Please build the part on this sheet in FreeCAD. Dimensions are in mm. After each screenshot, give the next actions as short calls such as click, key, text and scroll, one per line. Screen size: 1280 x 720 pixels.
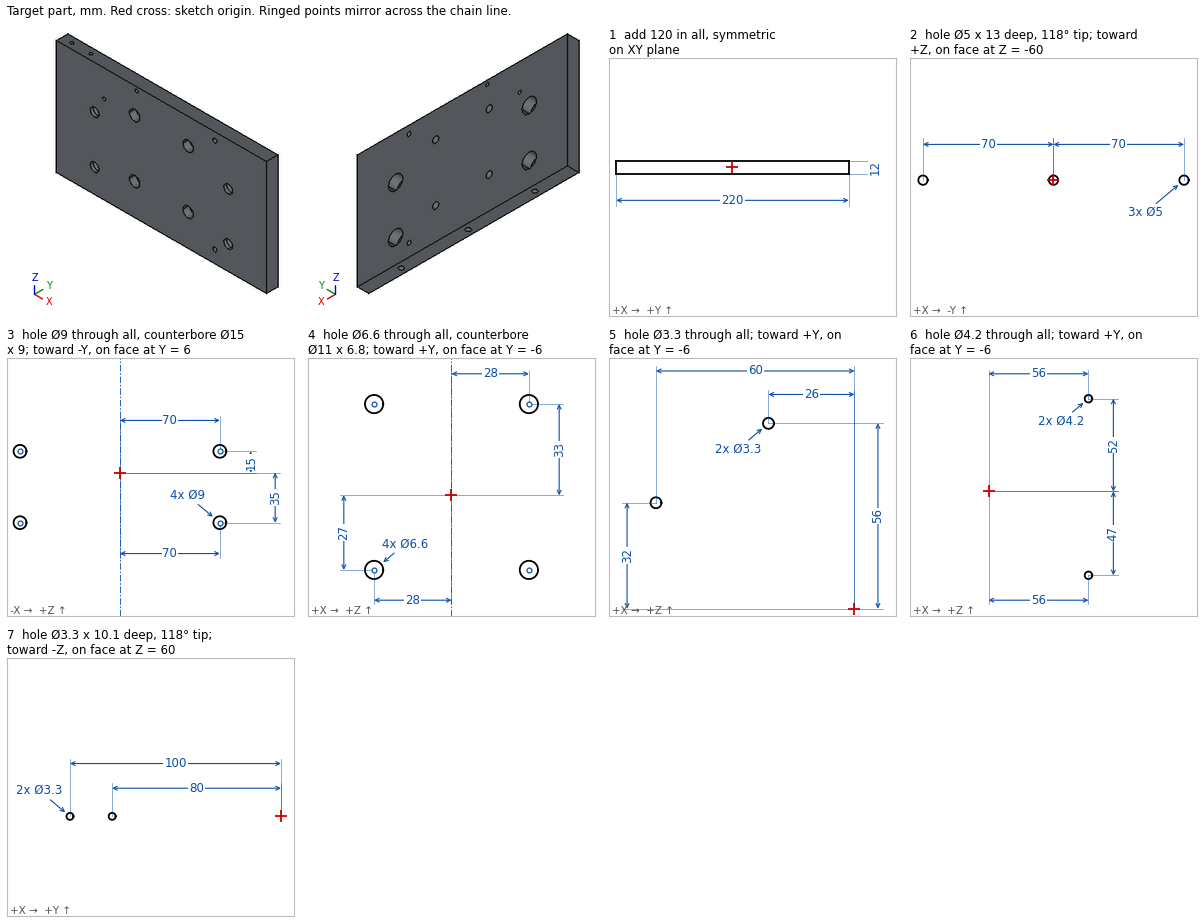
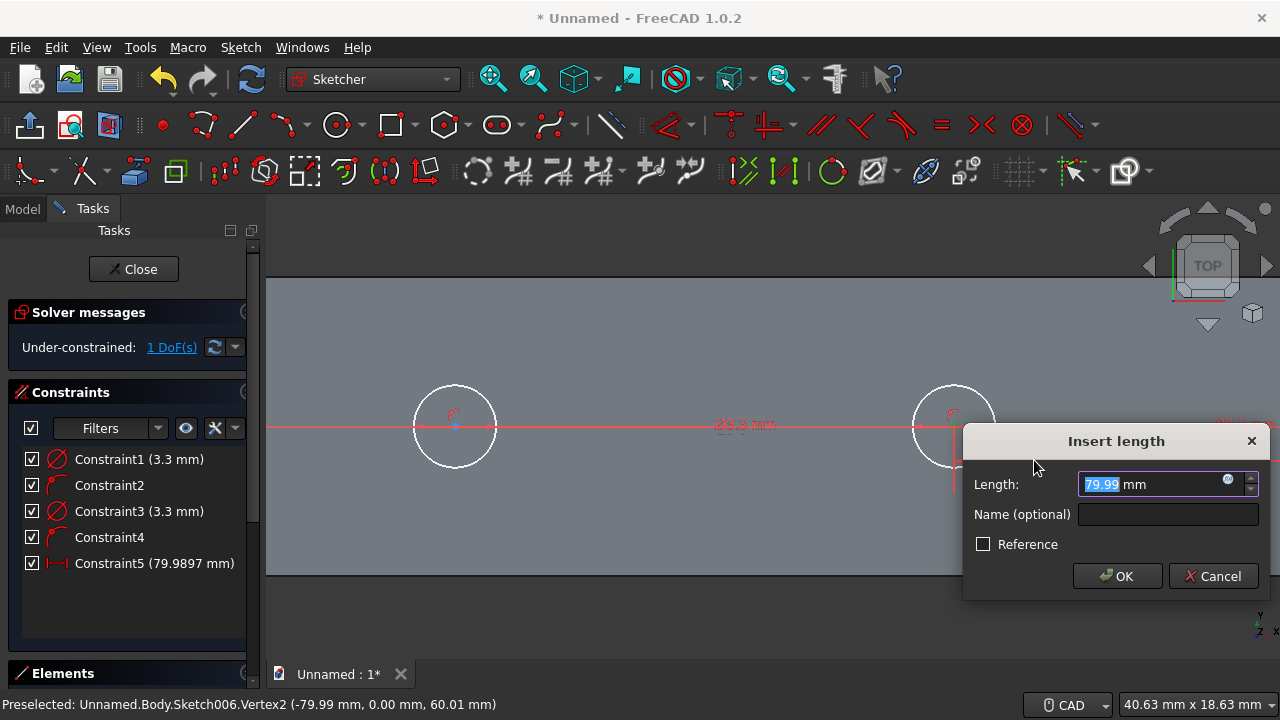
text(80)
key(Return)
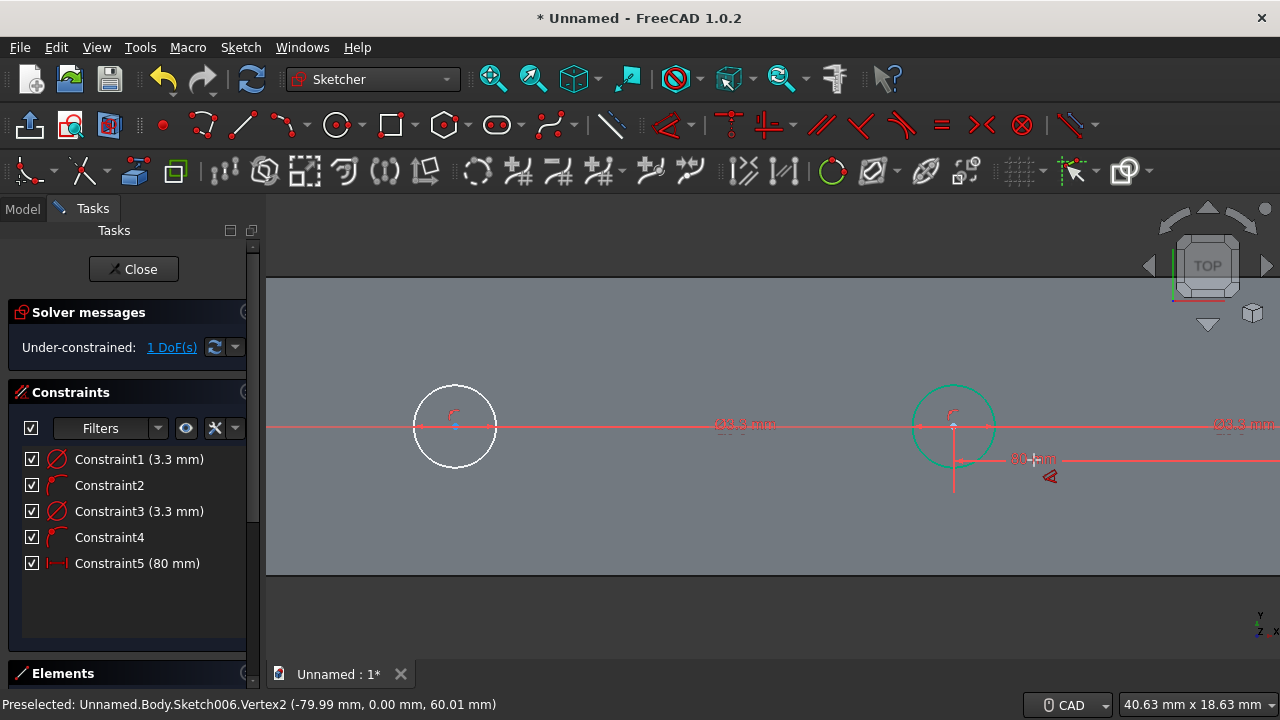
click(455, 426)
click(785, 460)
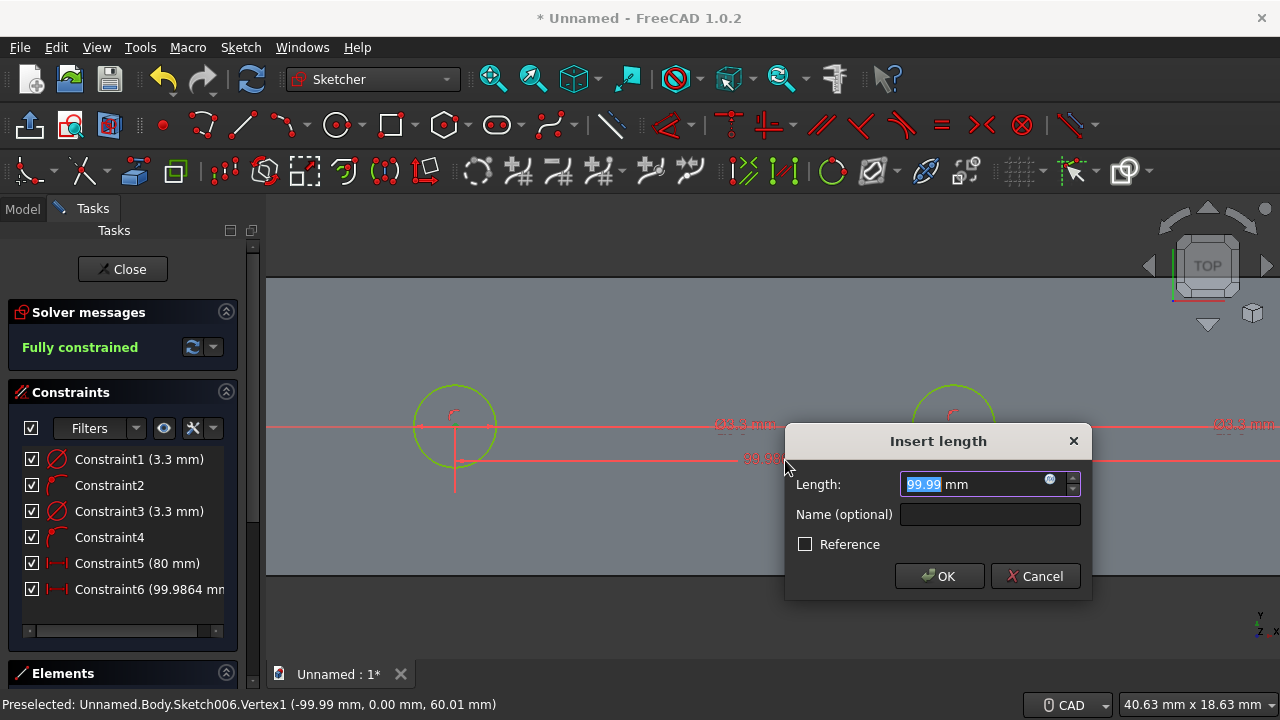
text(100)
key(Return)
key(Escape)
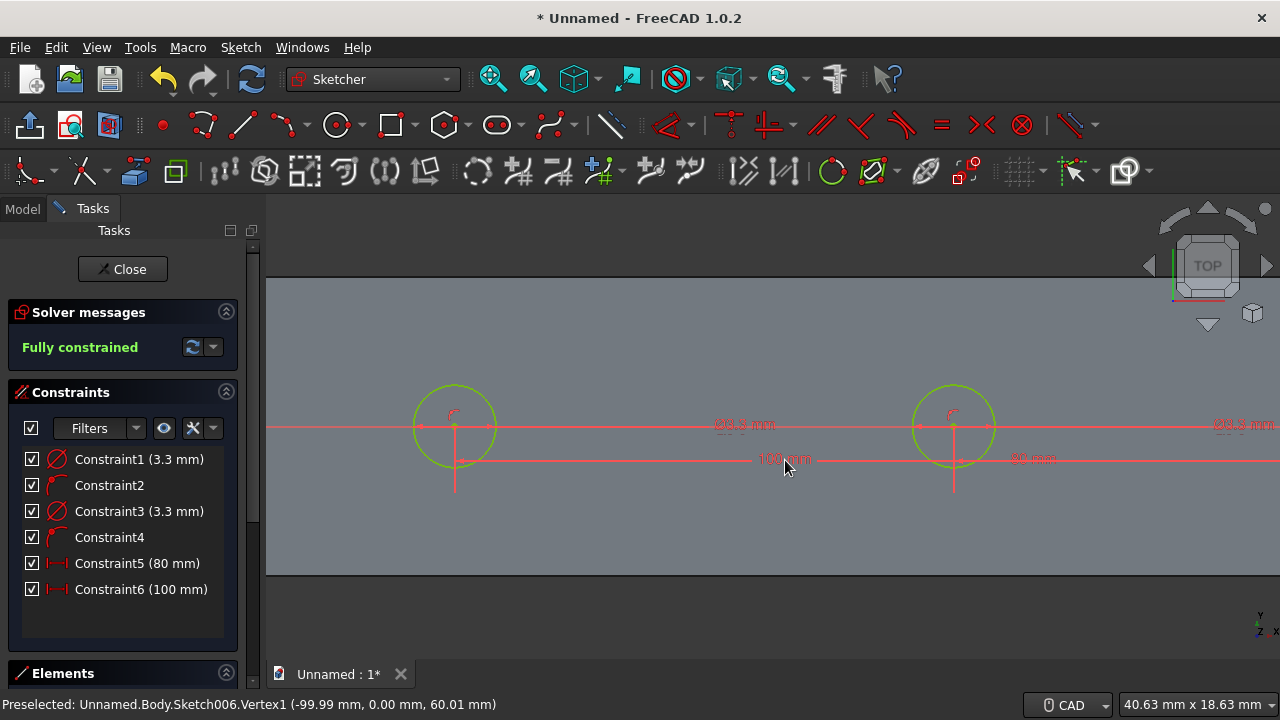
click(123, 269)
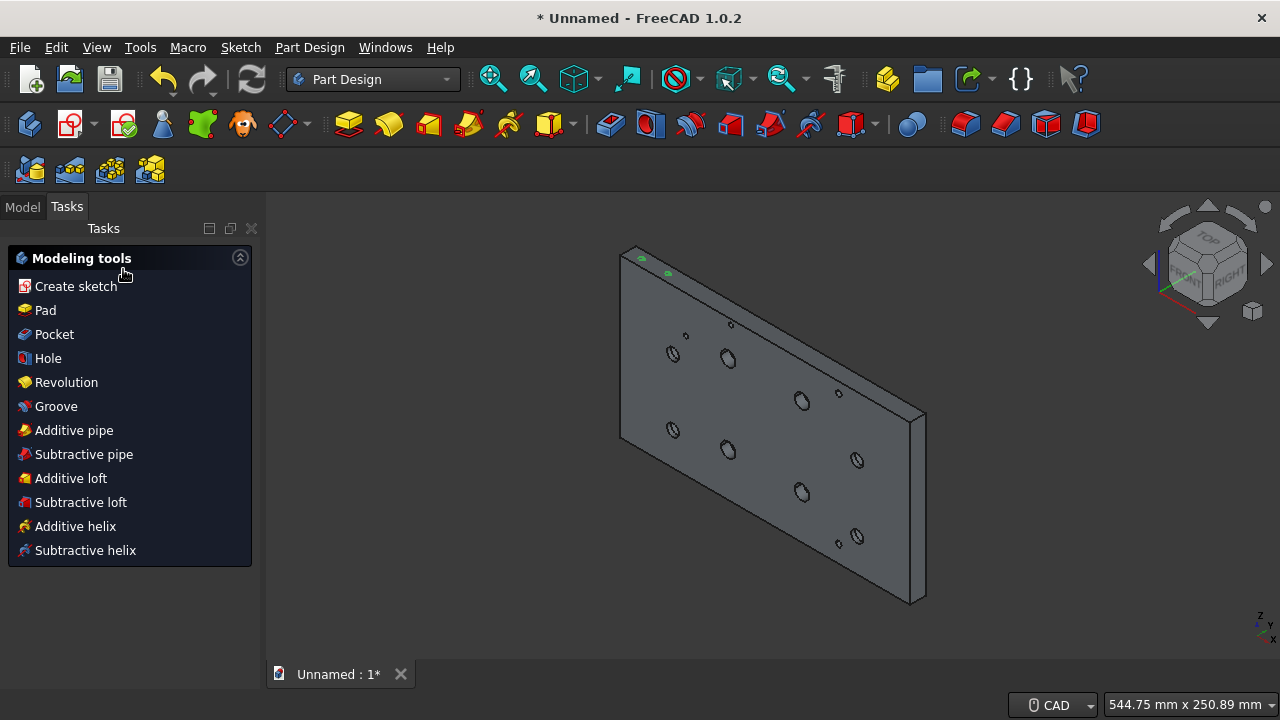
click(652, 124)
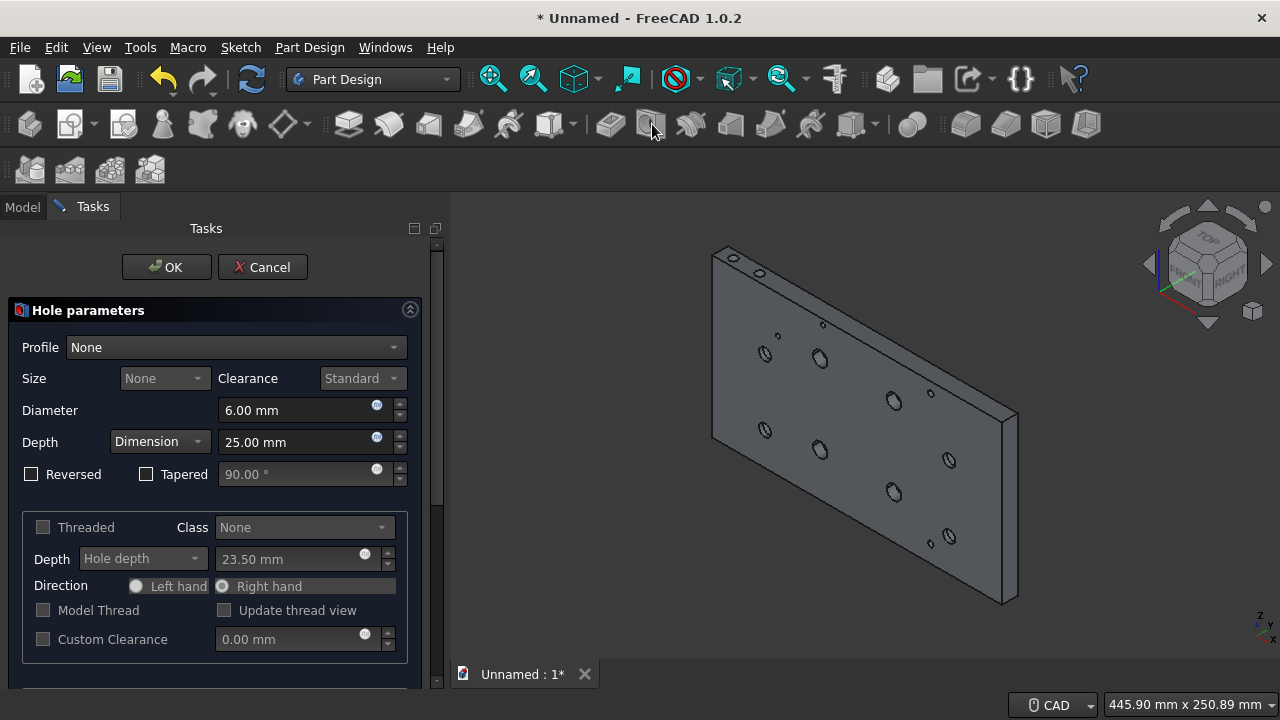
triple_click(305, 410)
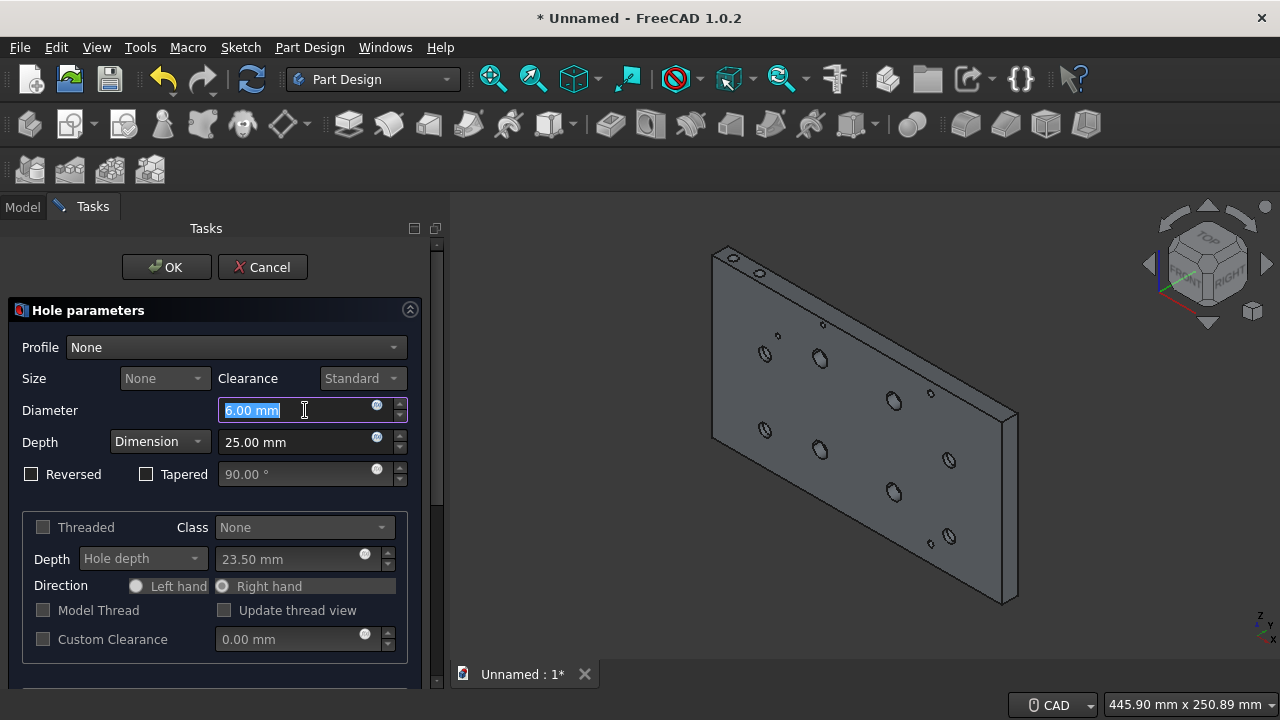
text(3.3)
key(Tab)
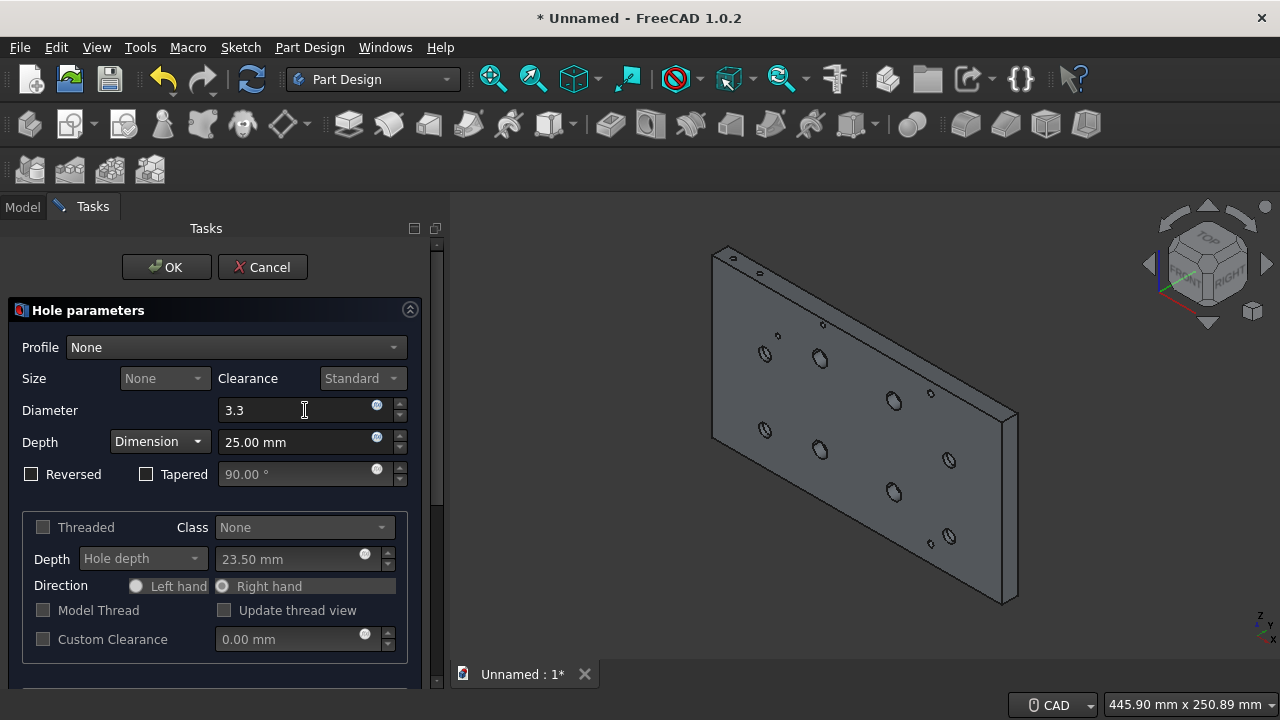
triple_click(305, 442)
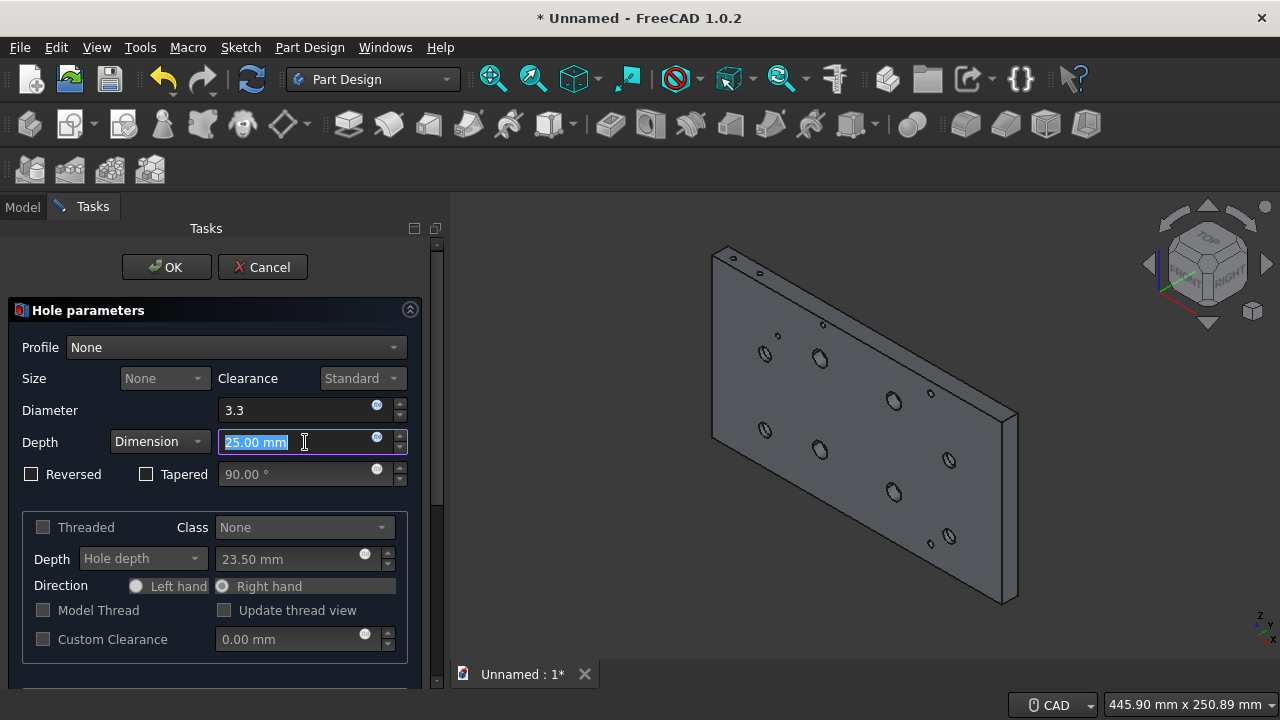
text(10.1)
key(Tab)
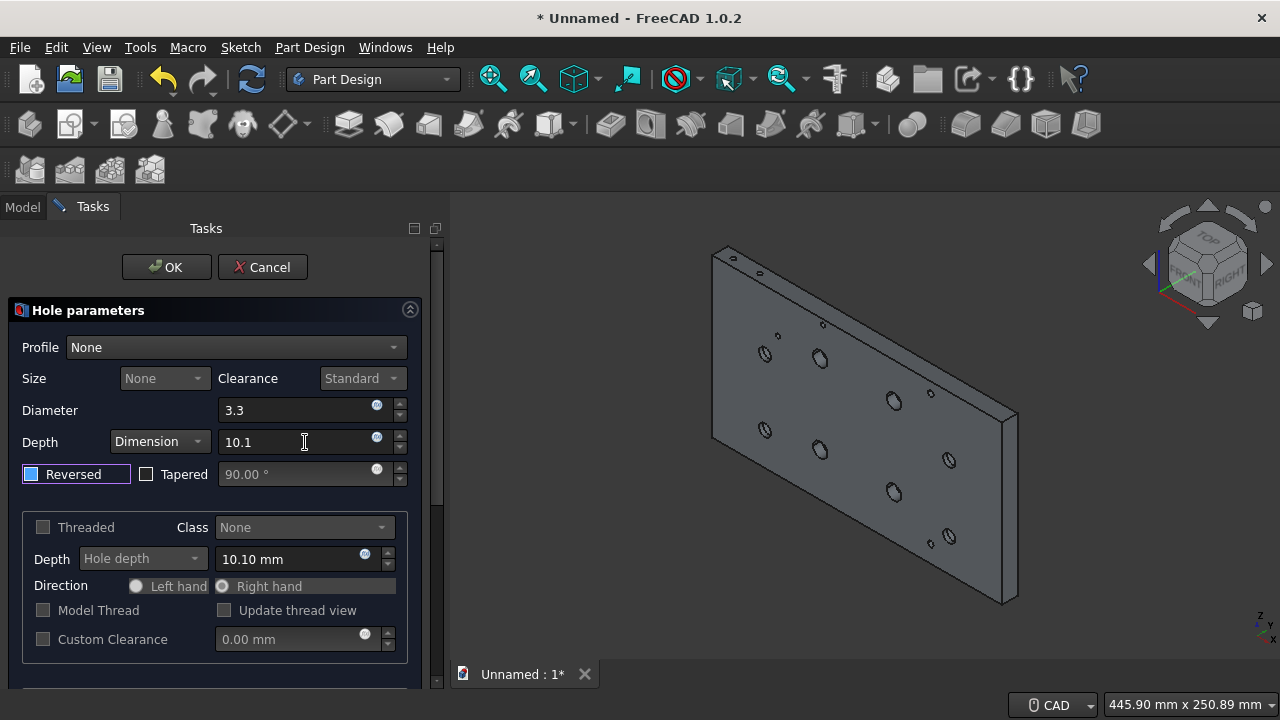
click(167, 267)